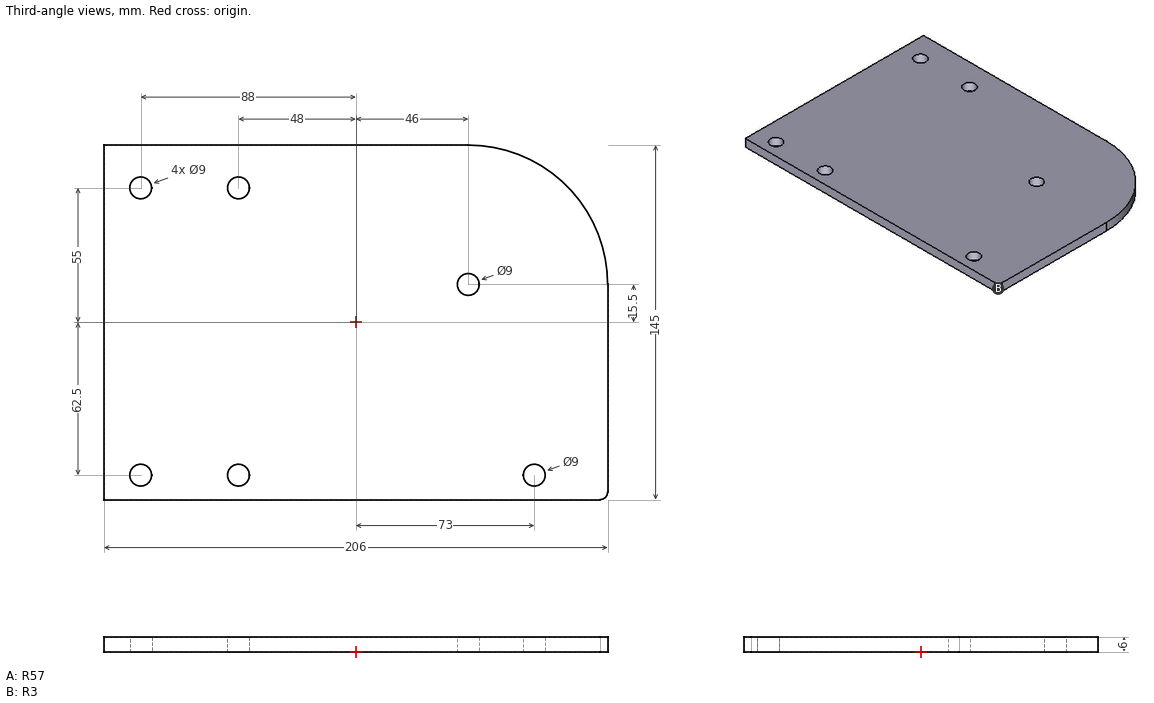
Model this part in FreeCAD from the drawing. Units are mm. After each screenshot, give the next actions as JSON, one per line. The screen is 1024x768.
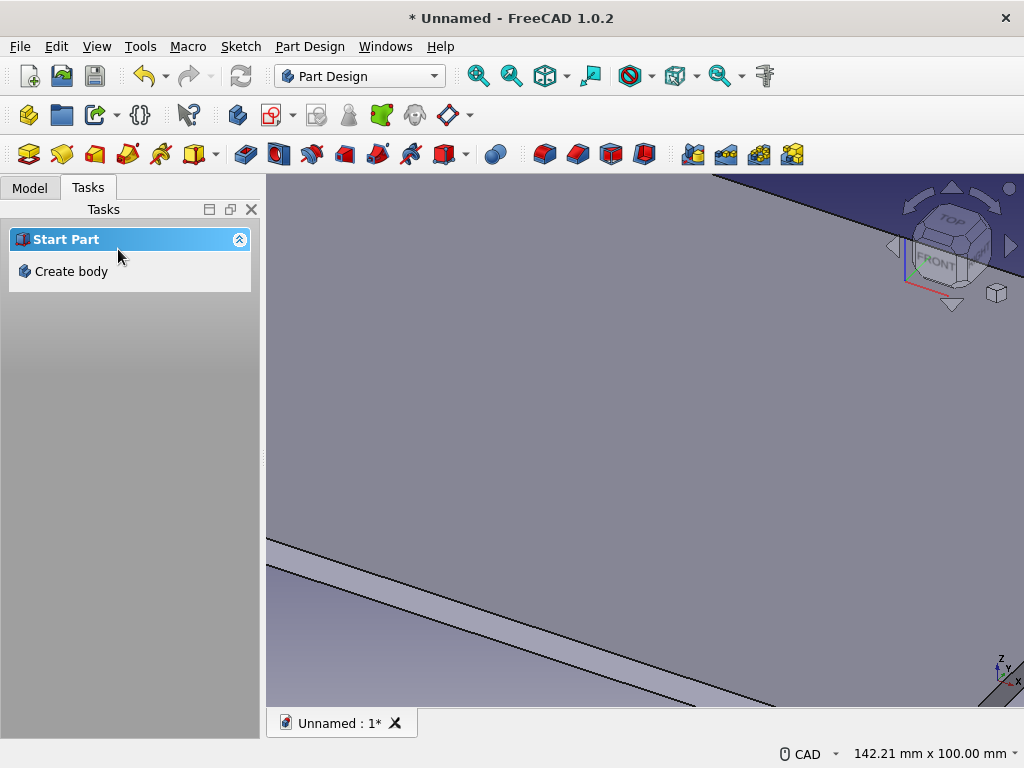
{"action": "key", "text": "v f"}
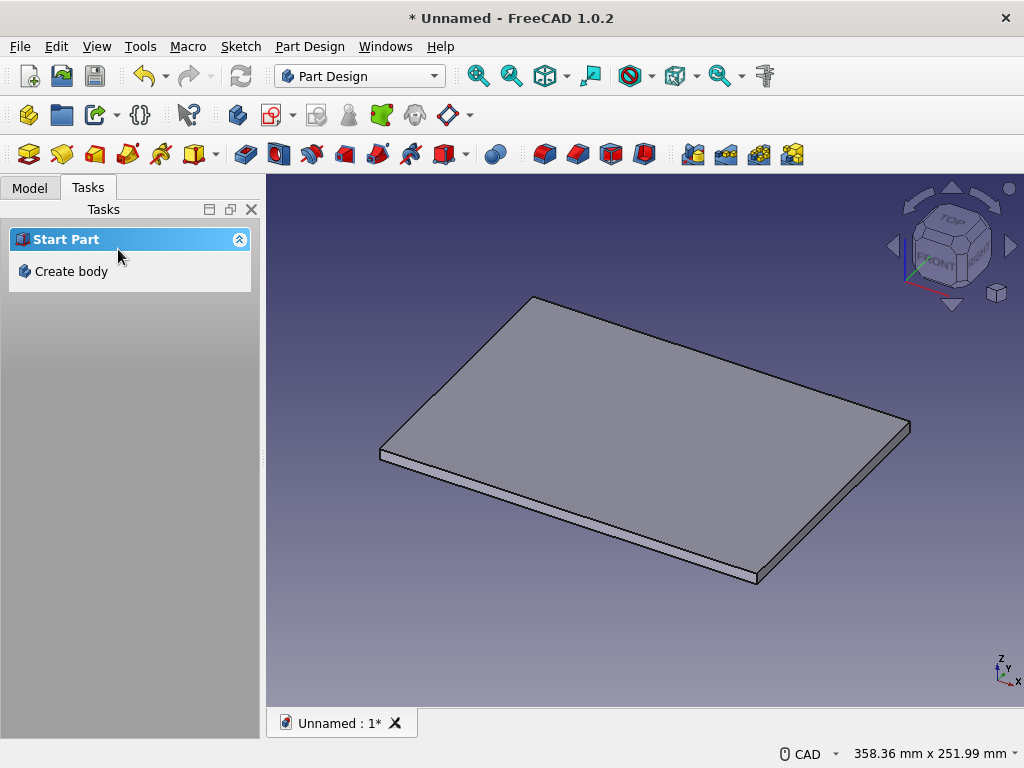
{"action": "left_click", "coordinate": [699, 452]}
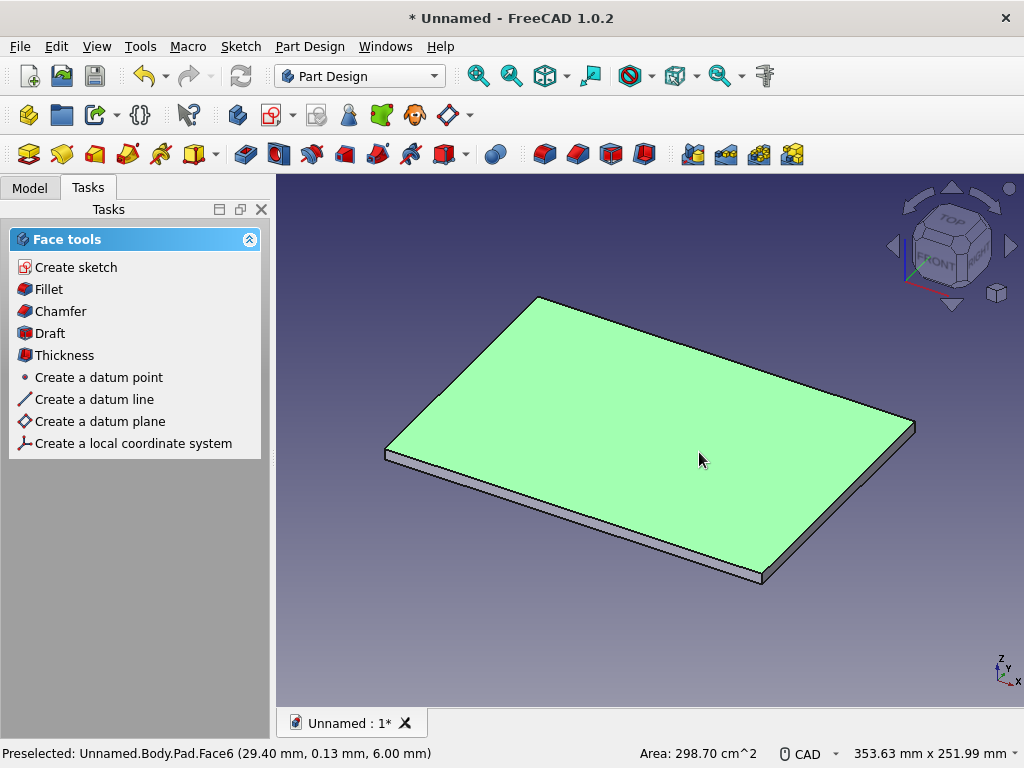
{"action": "left_click", "coordinate": [270, 116]}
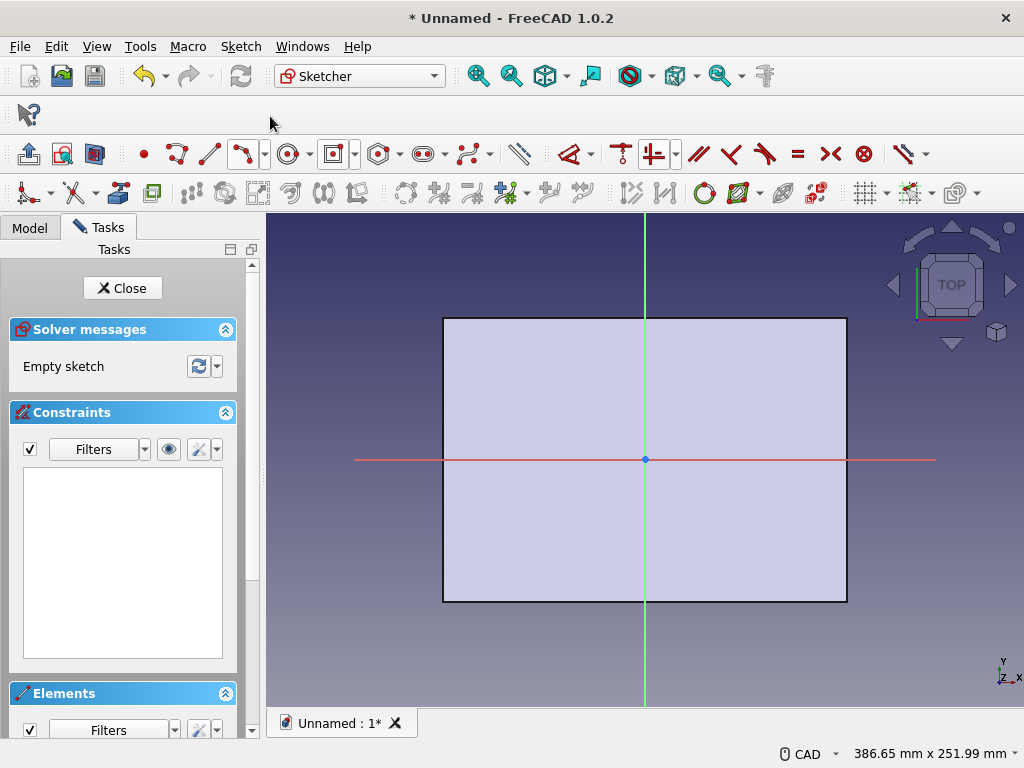
{"action": "key", "text": "g c"}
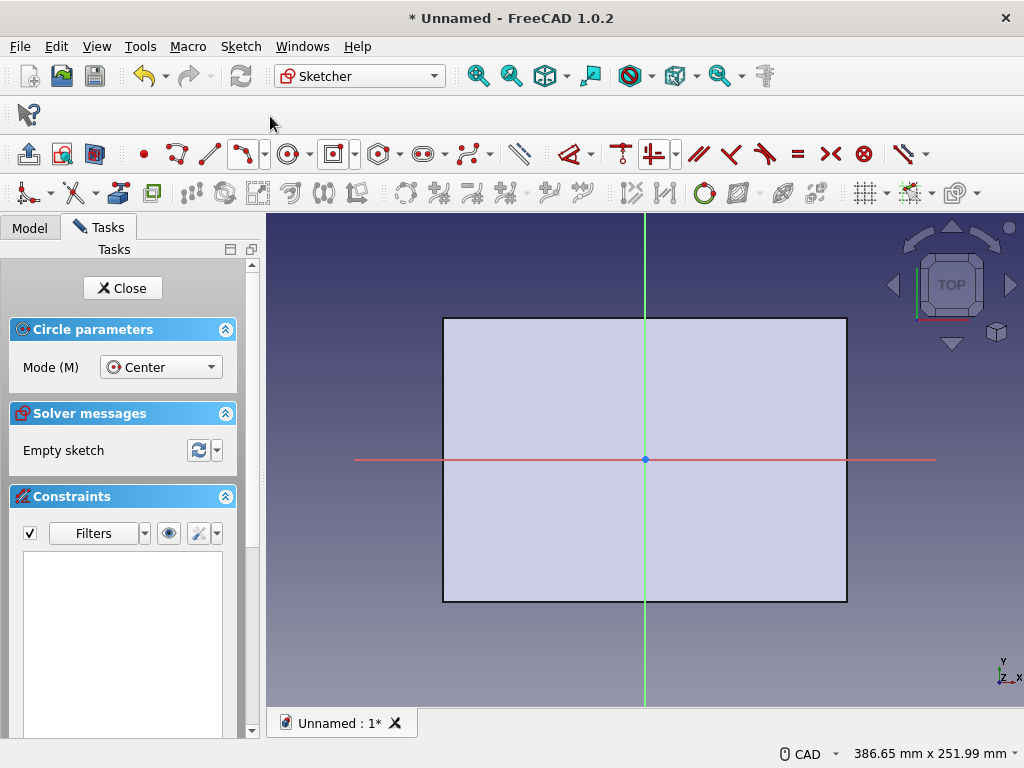
{"action": "scroll", "coordinate": [472, 352], "scroll_direction": "up", "scroll_amount": 5}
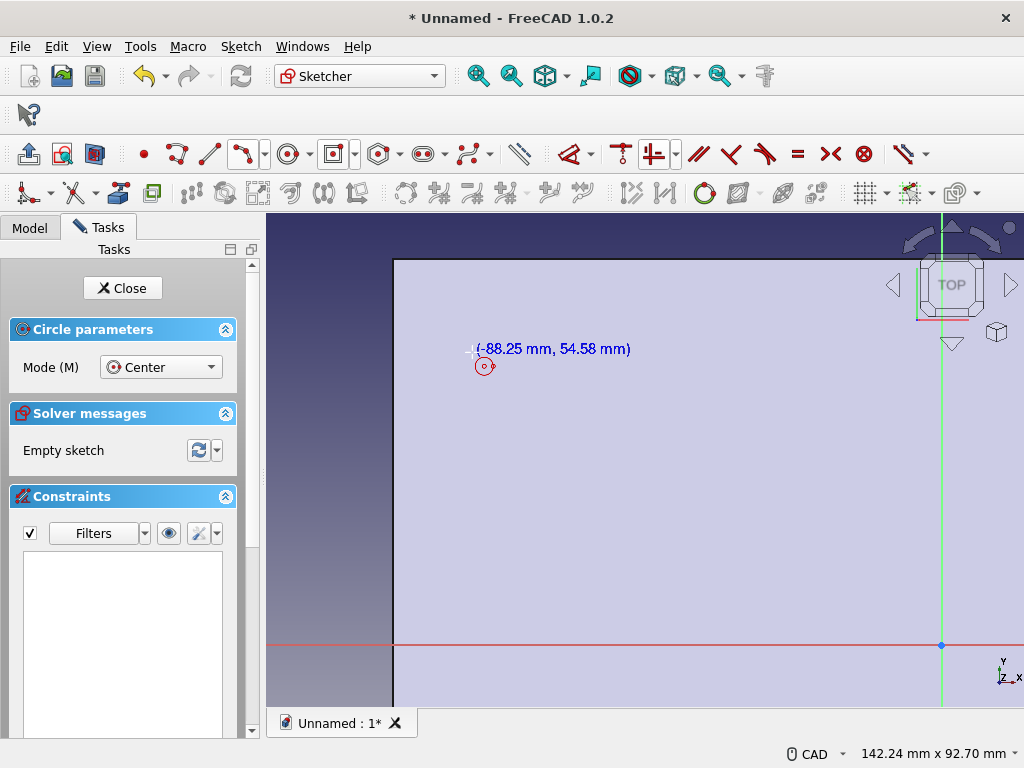
{"action": "left_click", "coordinate": [473, 352]}
{"action": "mouse_move", "coordinate": [490, 335]}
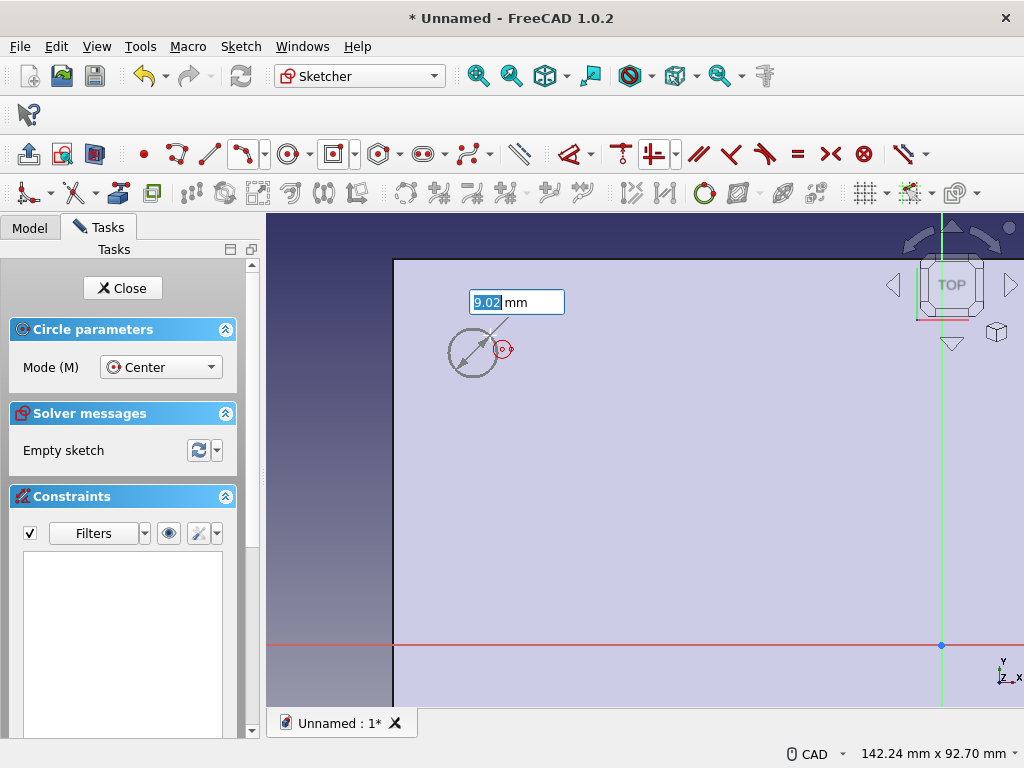
{"action": "type", "text": "9"}
{"action": "key", "text": "Return"}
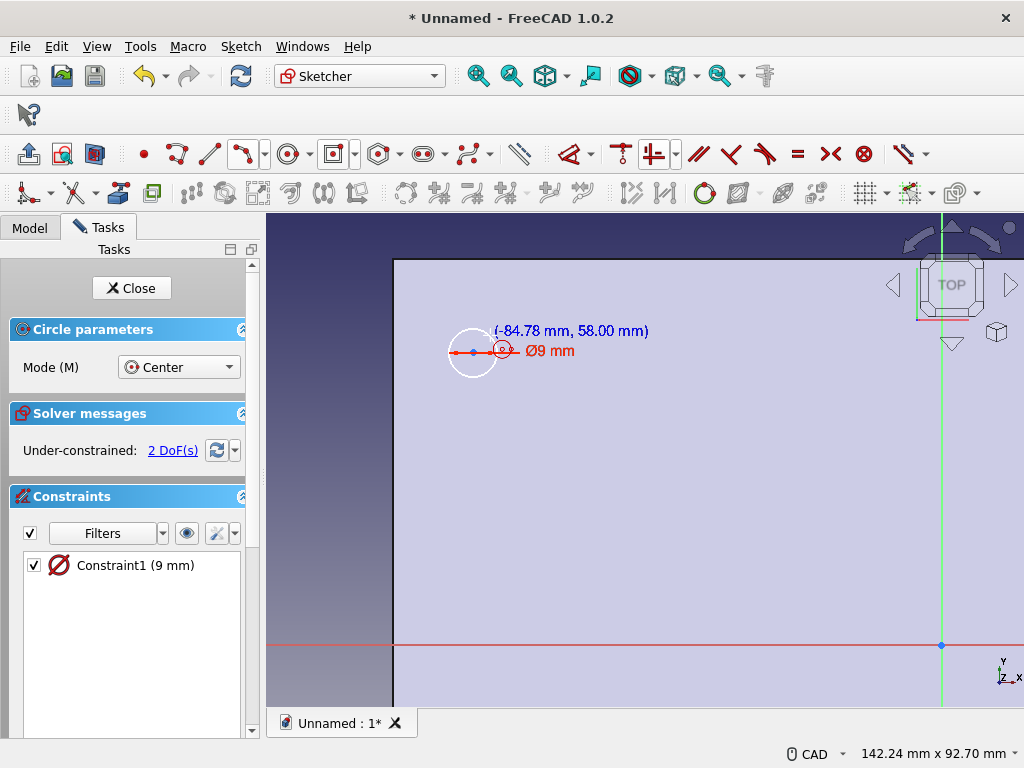
{"action": "left_click", "coordinate": [686, 352]}
{"action": "mouse_move", "coordinate": [703, 335]}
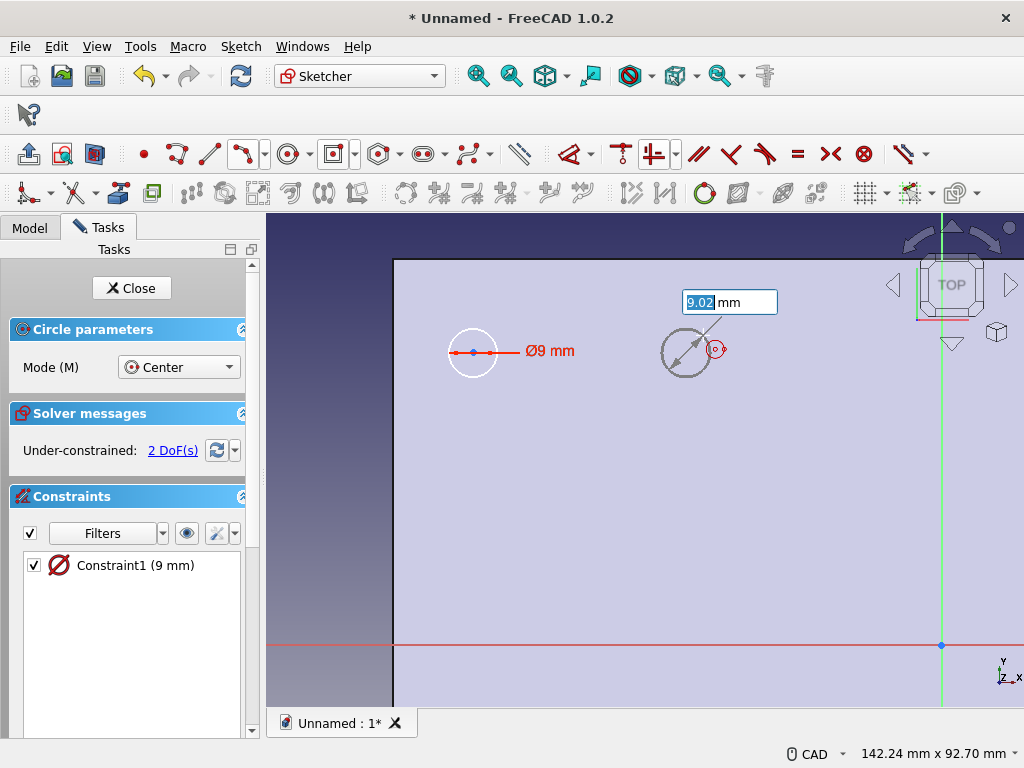
{"action": "type", "text": "9"}
{"action": "key", "text": "Return"}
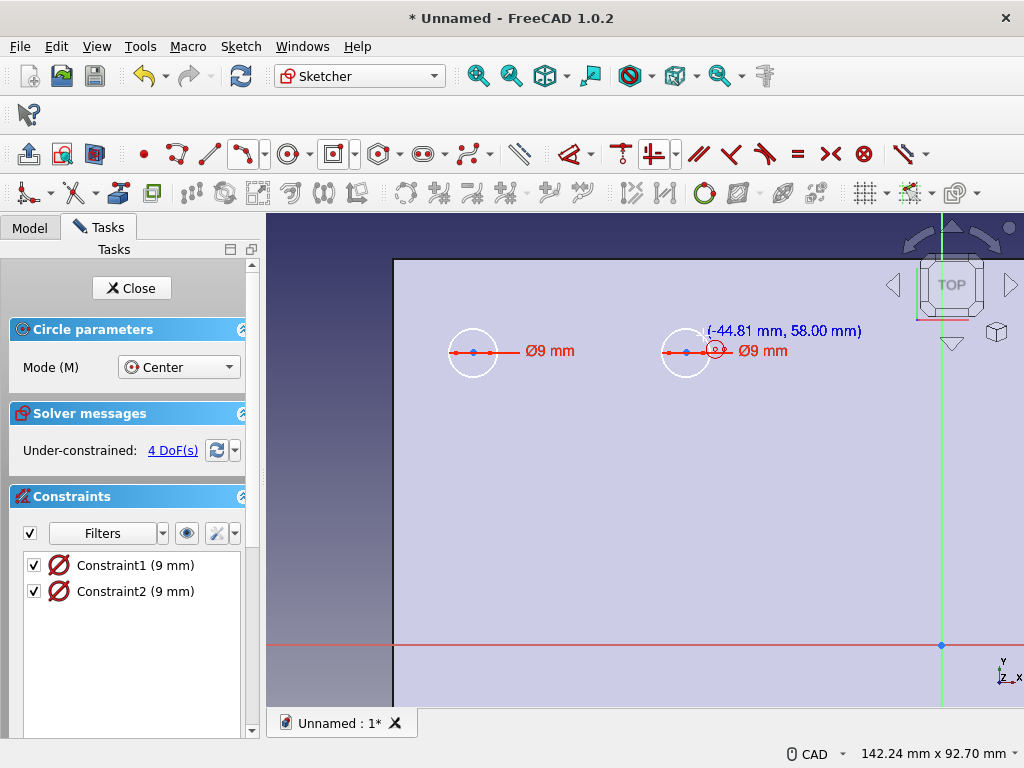
{"action": "scroll", "coordinate": [480, 293], "scroll_direction": "down", "scroll_amount": 4}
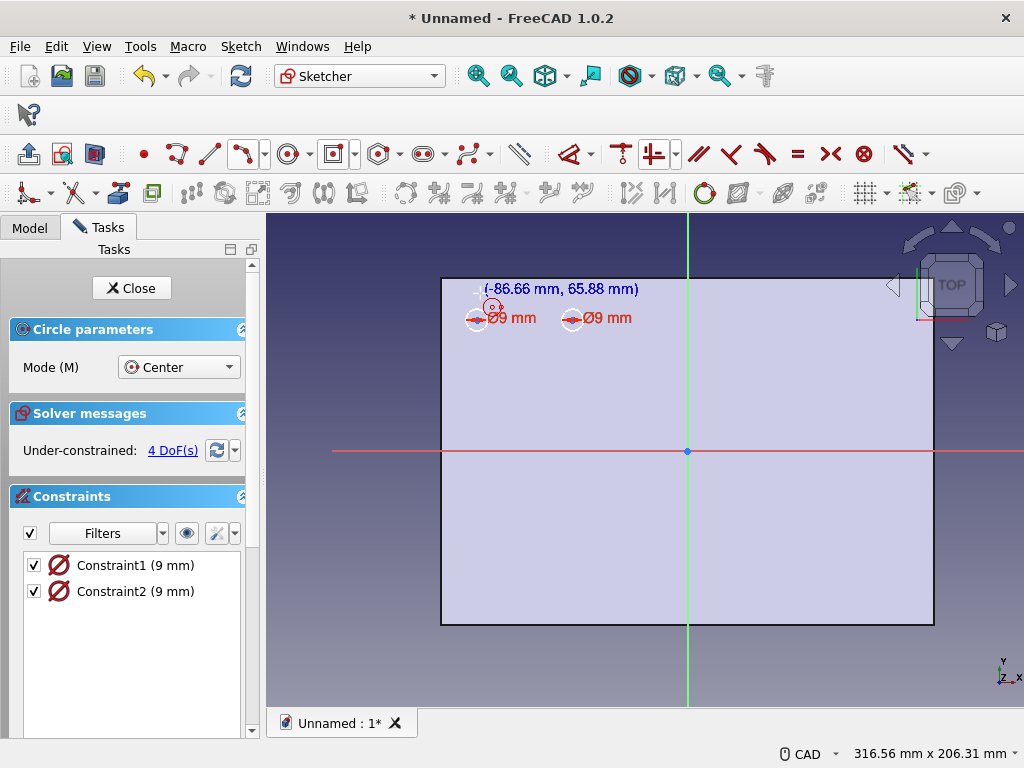
{"action": "scroll", "coordinate": [477, 601], "scroll_direction": "up", "scroll_amount": 4}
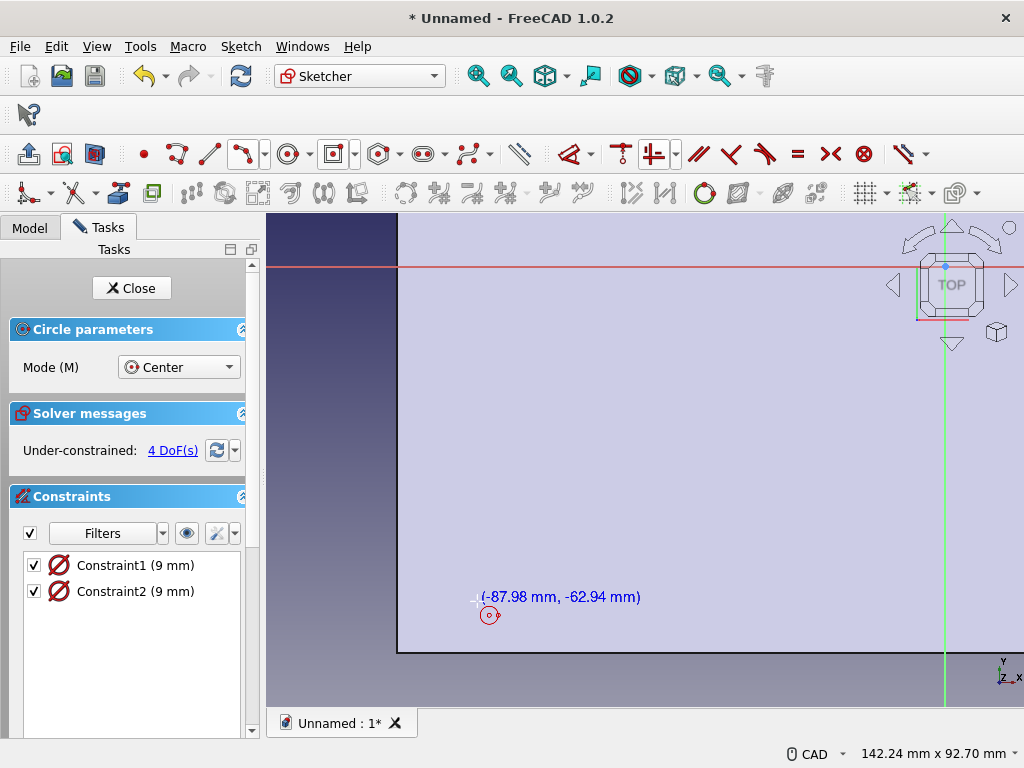
{"action": "left_click", "coordinate": [477, 600]}
{"action": "mouse_move", "coordinate": [493, 583]}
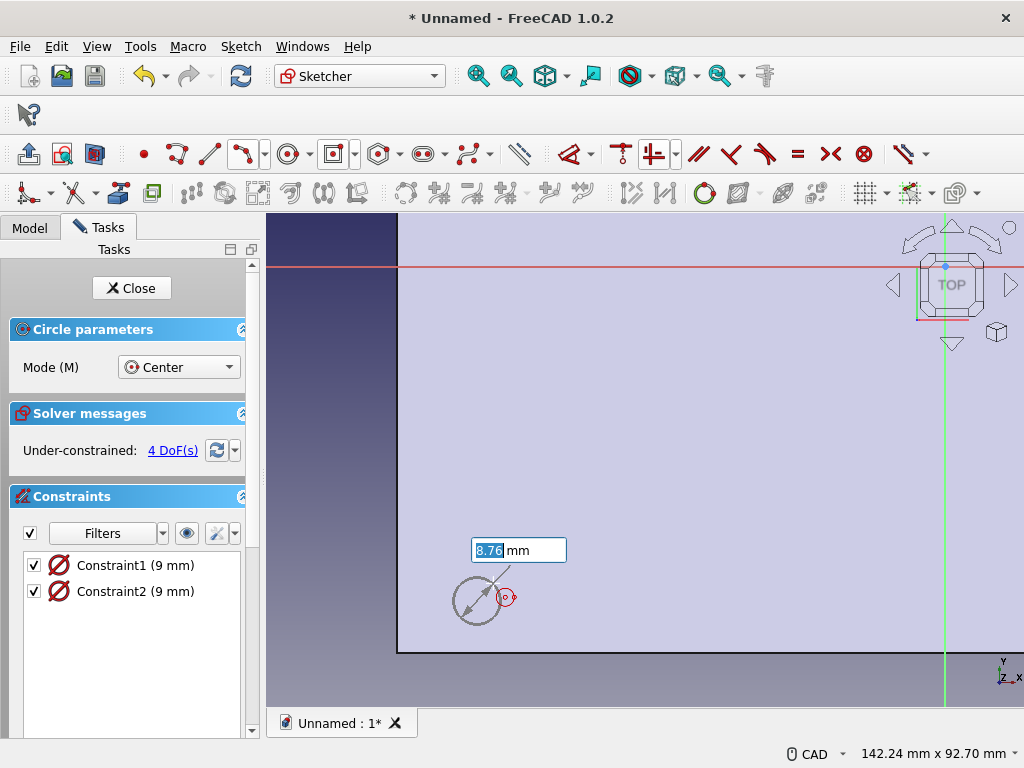
{"action": "type", "text": "9"}
{"action": "key", "text": "Return"}